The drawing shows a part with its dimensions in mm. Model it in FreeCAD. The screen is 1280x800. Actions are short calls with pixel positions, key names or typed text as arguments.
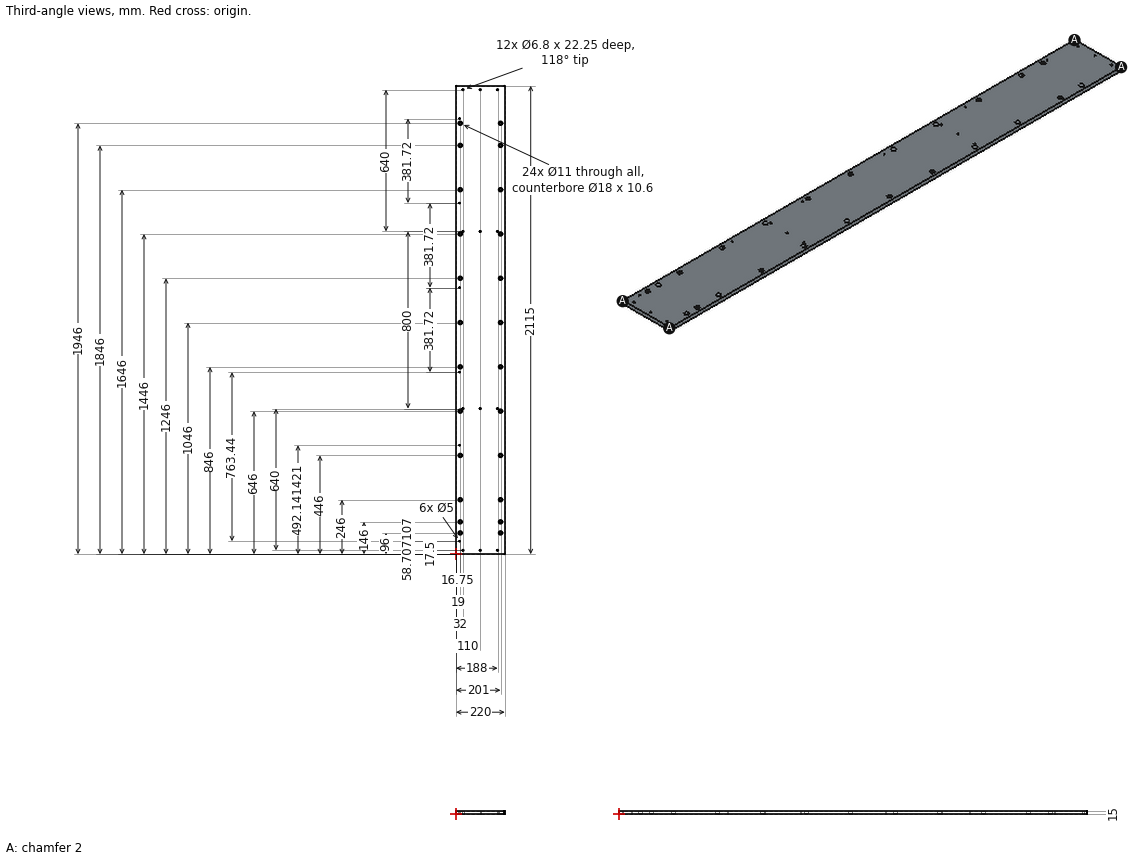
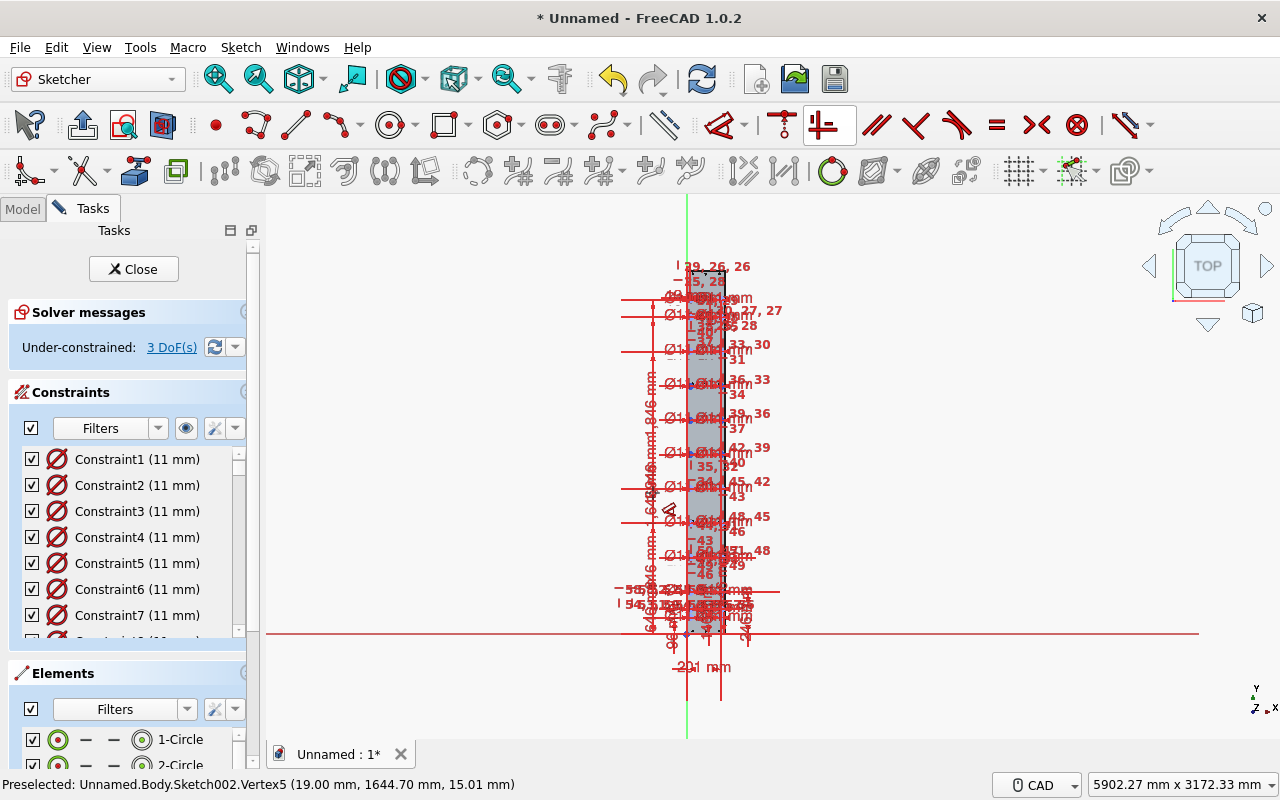
click(690, 386)
click(653, 423)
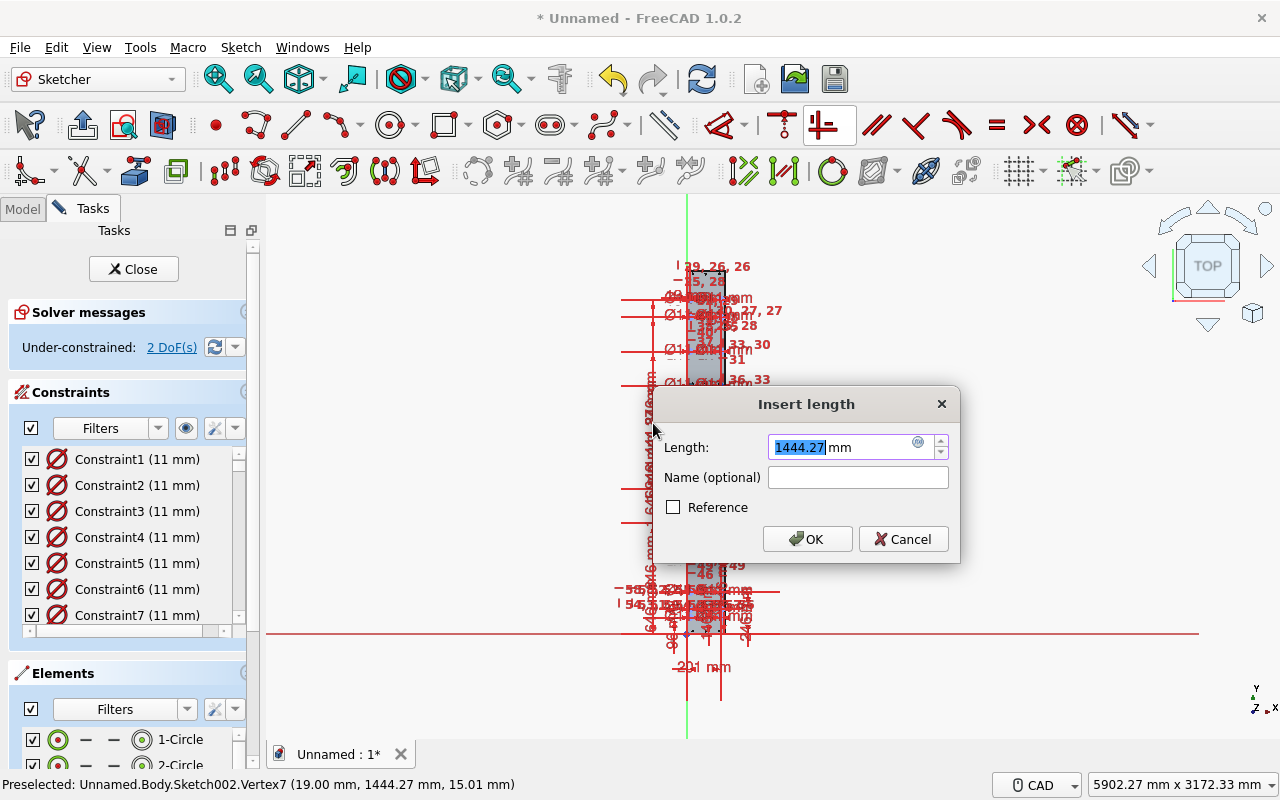
text(1446)
key(Return)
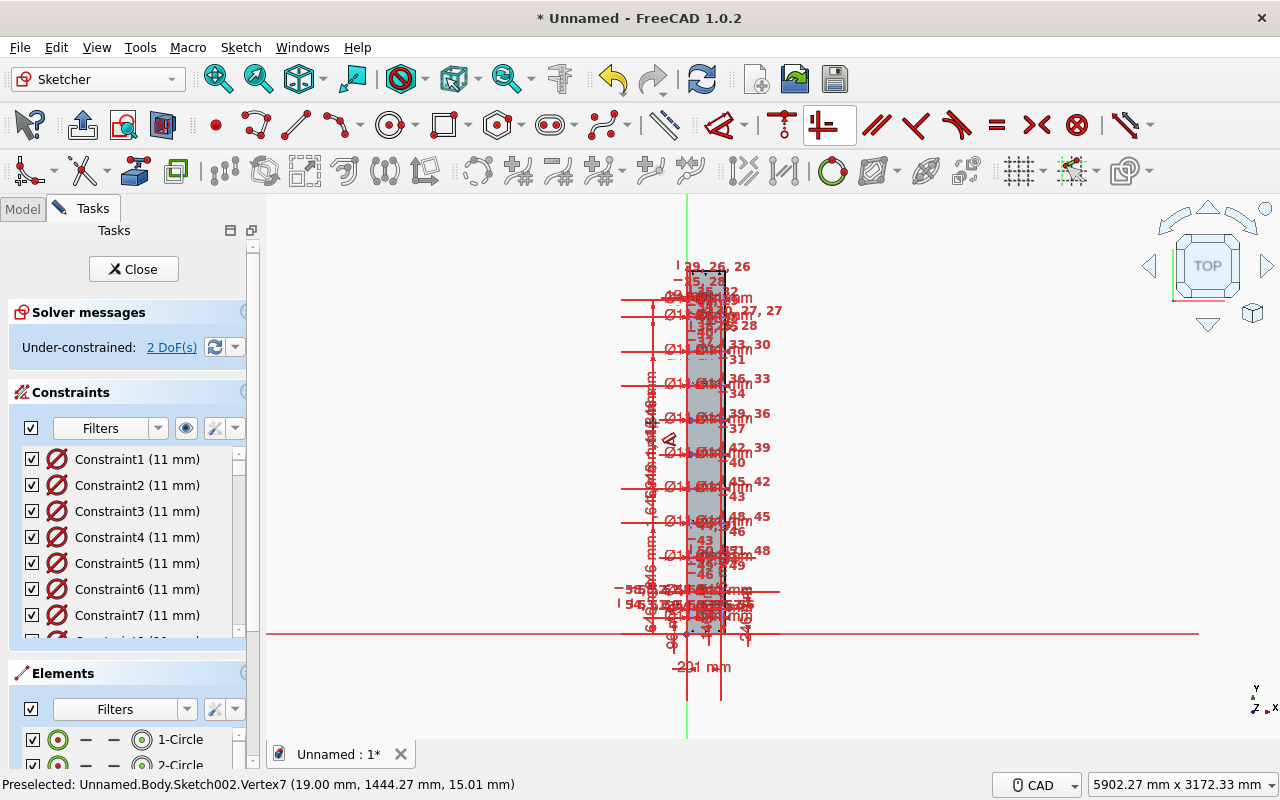
click(690, 420)
click(653, 527)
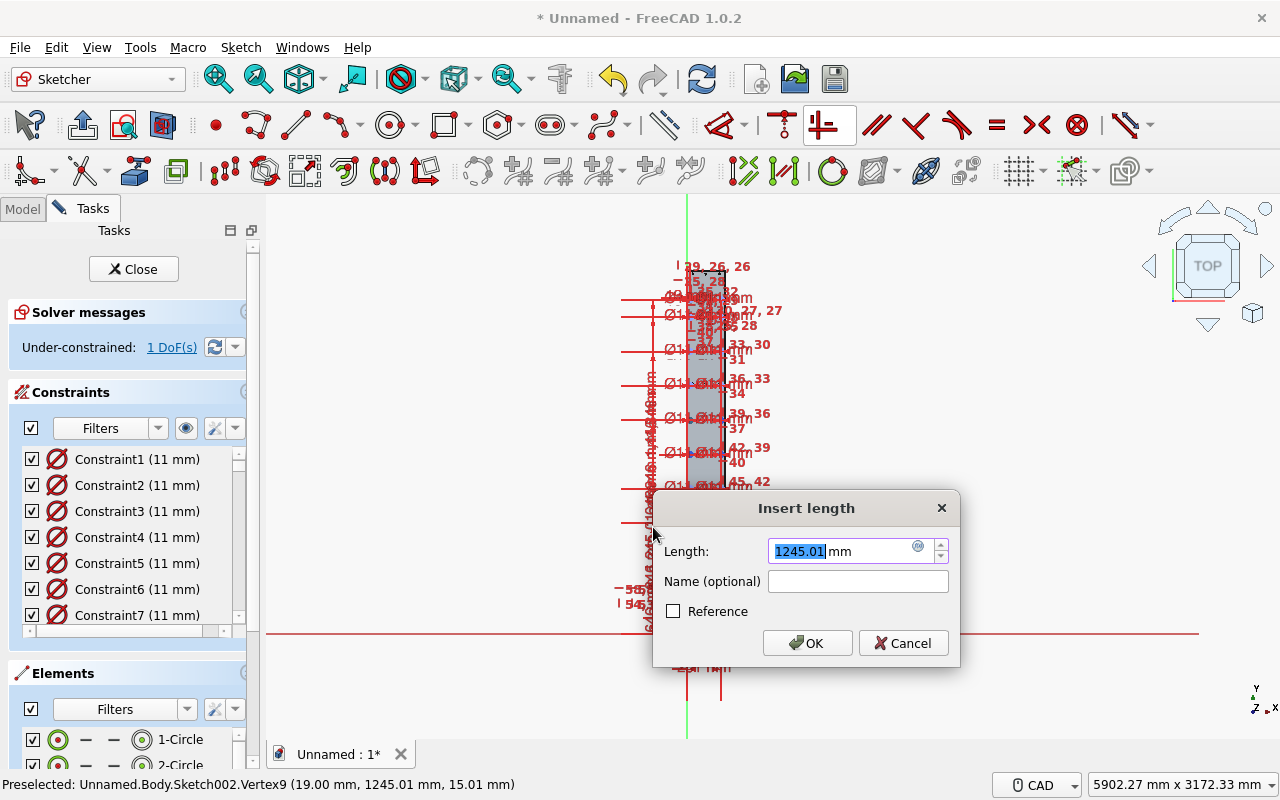
text(1246)
key(Return)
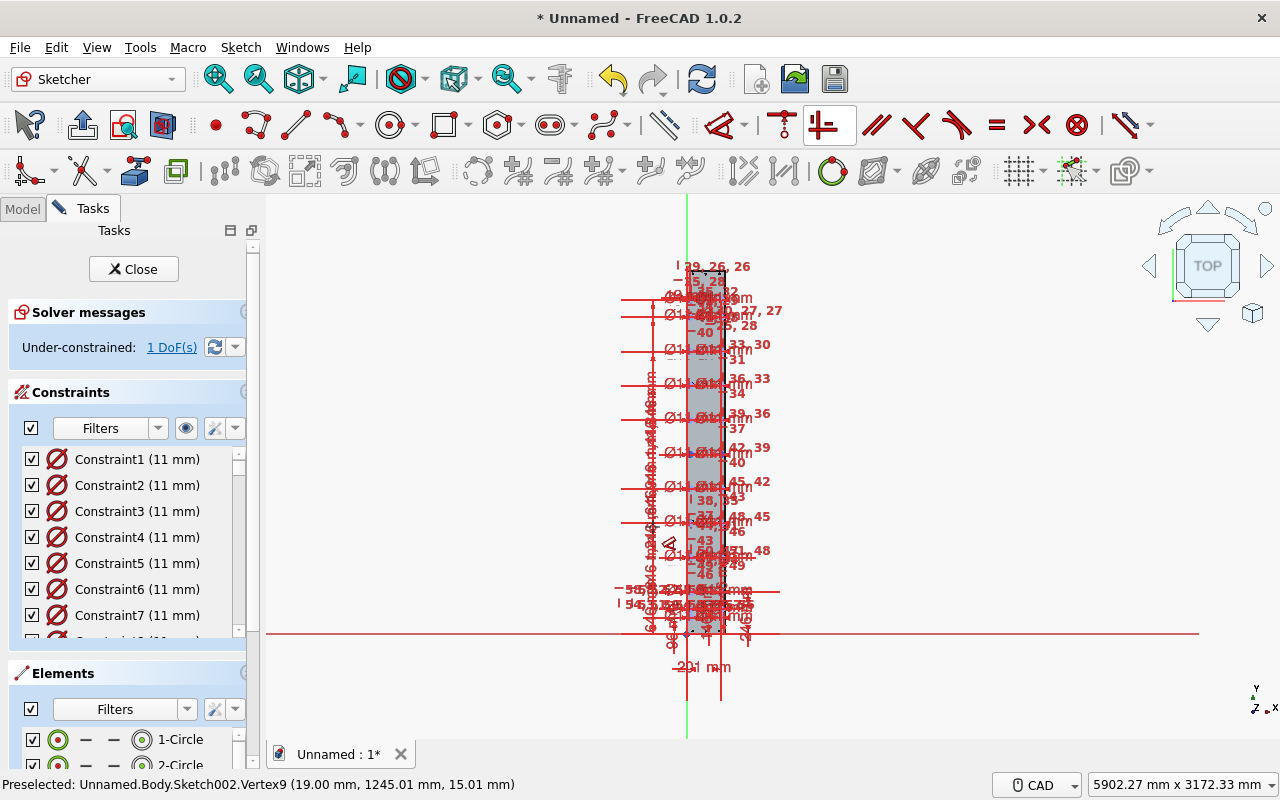
click(690, 455)
click(724, 503)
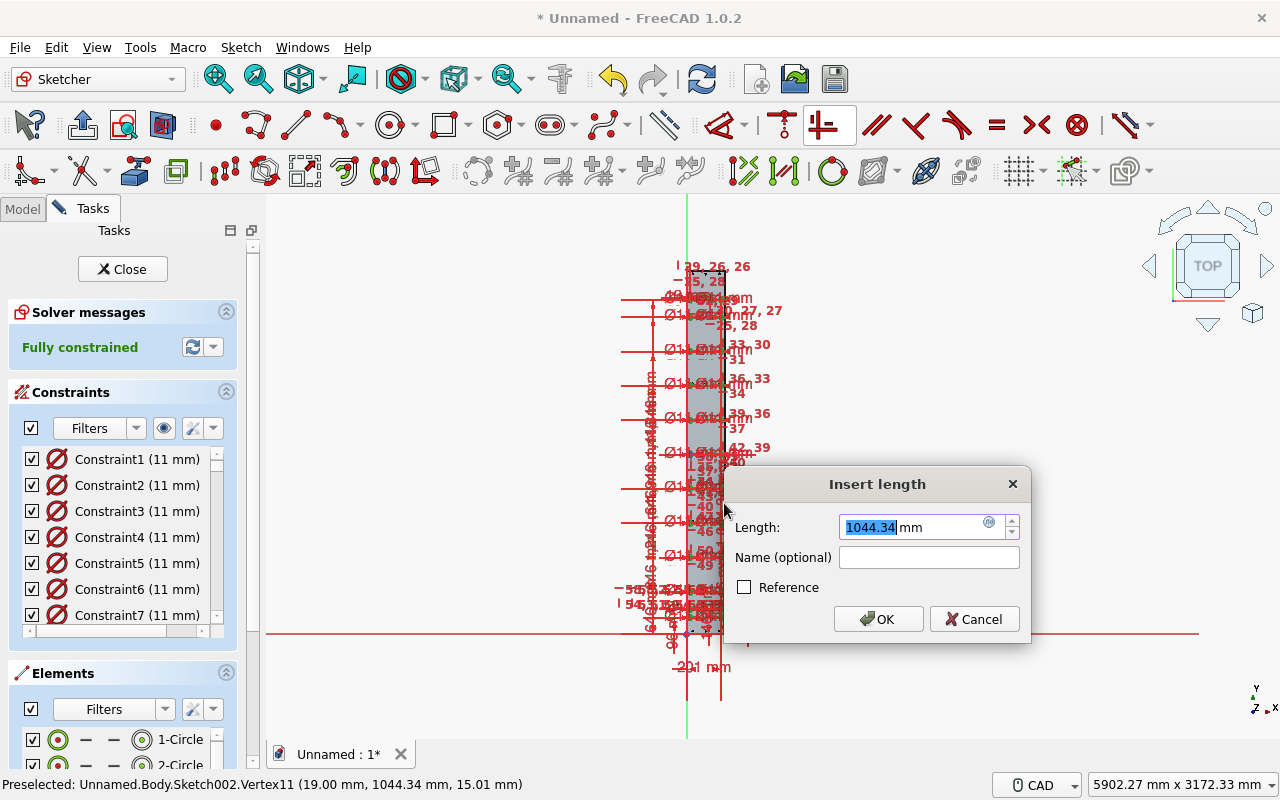
text(1046)
key(Return)
key(Escape)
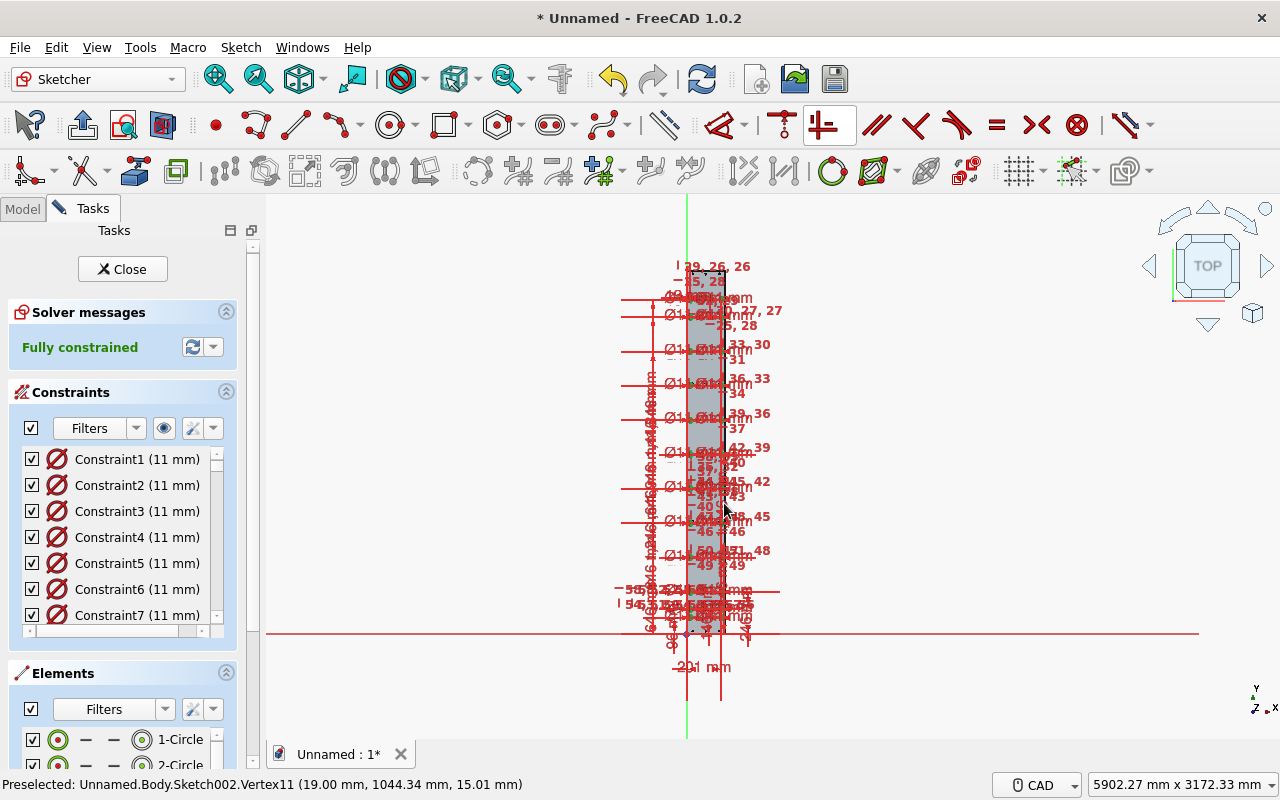
click(123, 269)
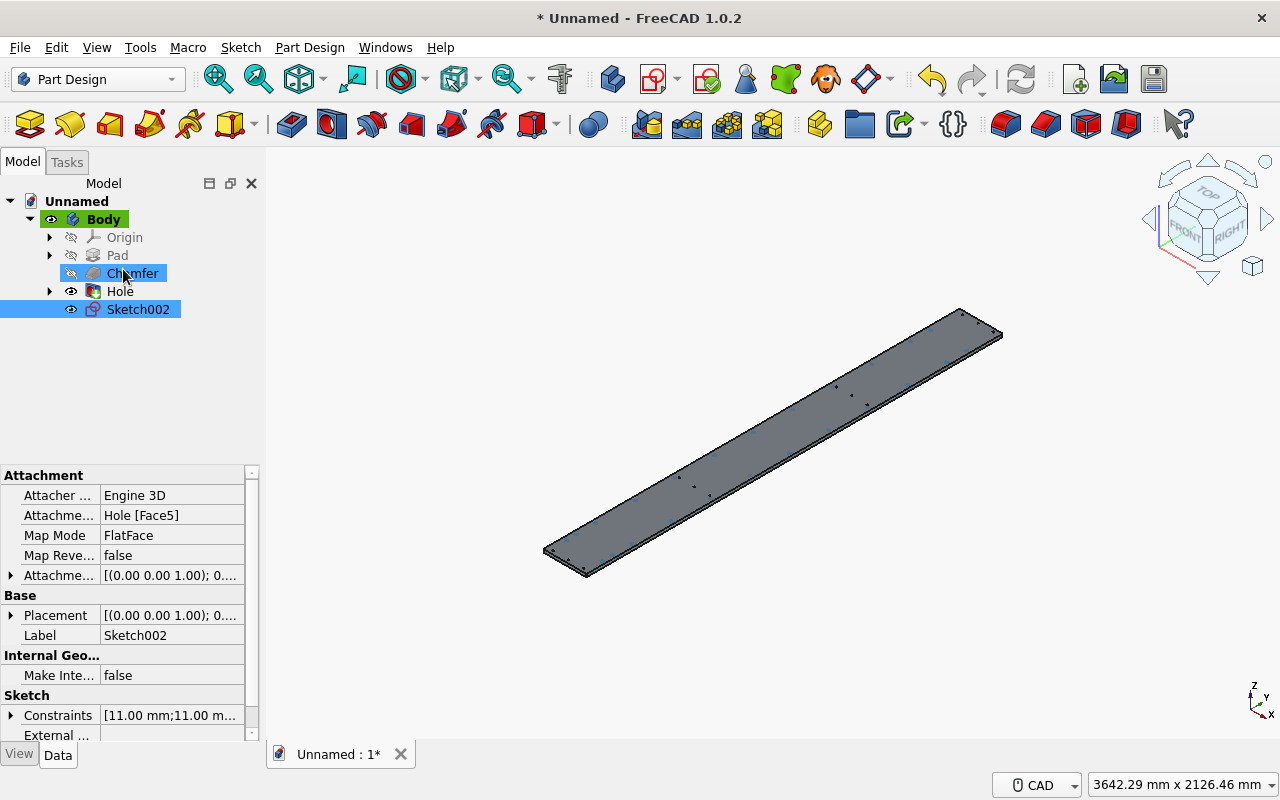
click(332, 124)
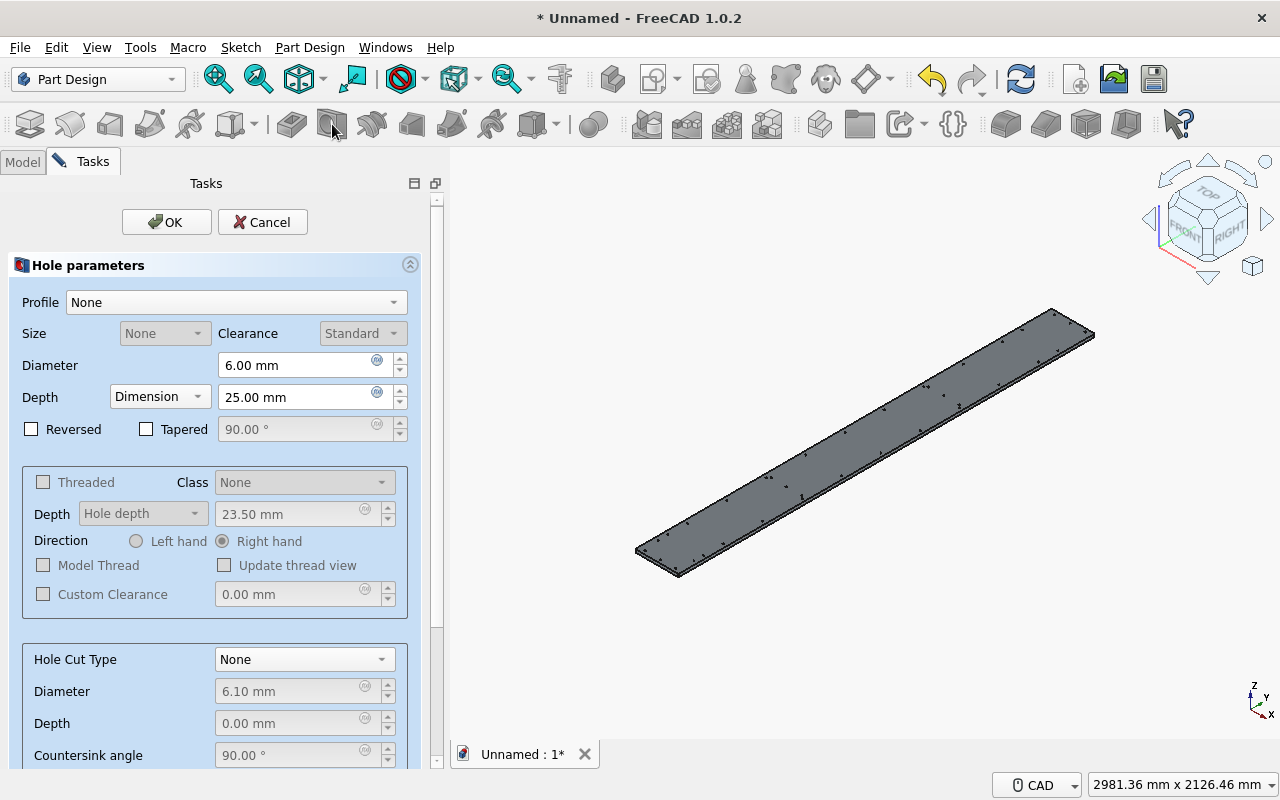
triple_click(305, 365)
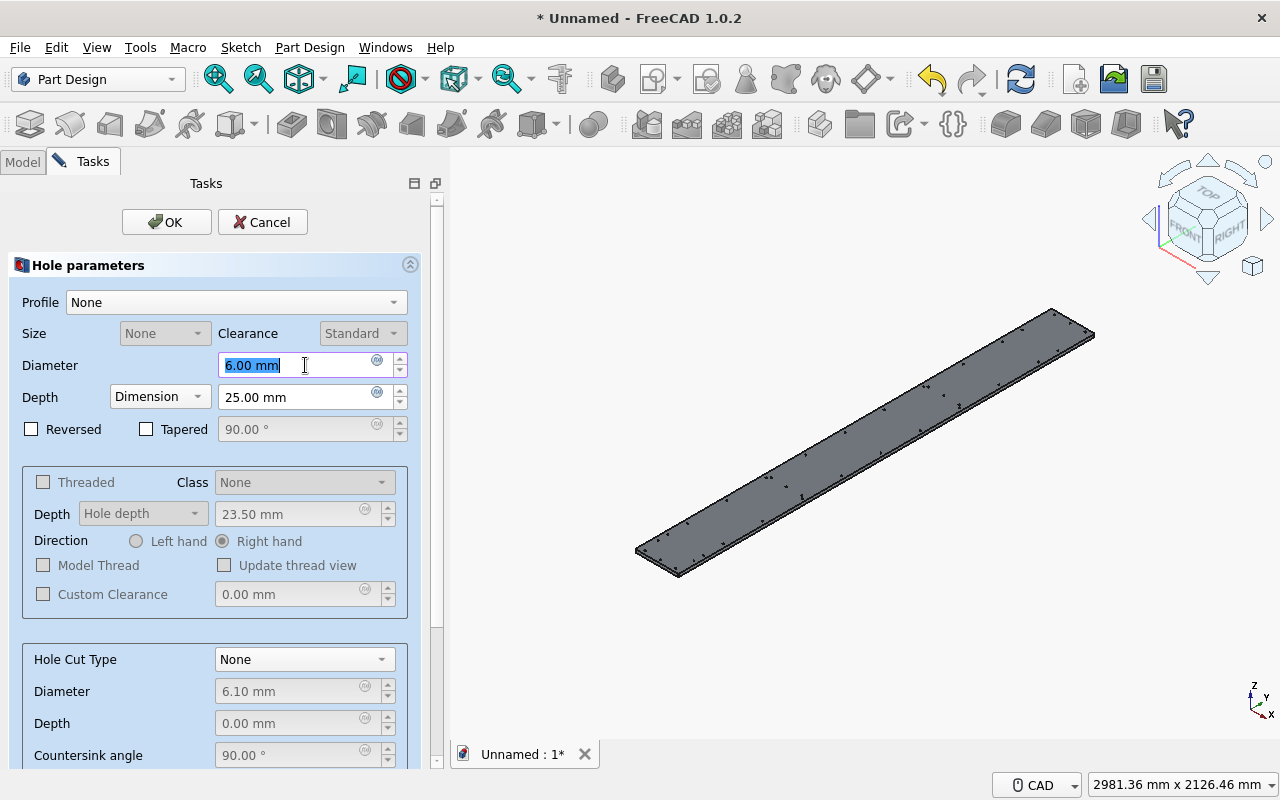
text(11)
key(Tab)